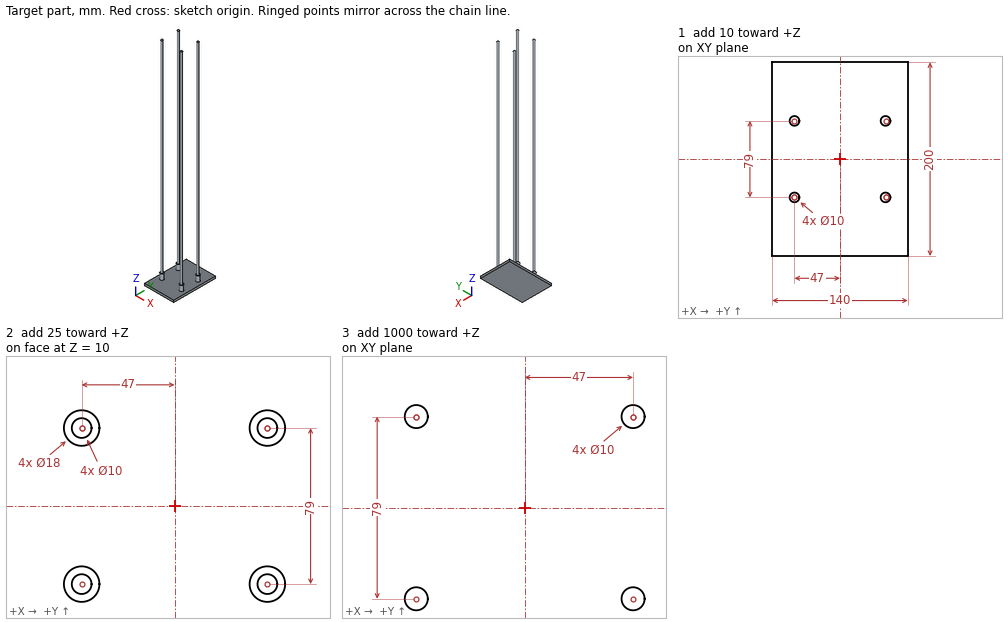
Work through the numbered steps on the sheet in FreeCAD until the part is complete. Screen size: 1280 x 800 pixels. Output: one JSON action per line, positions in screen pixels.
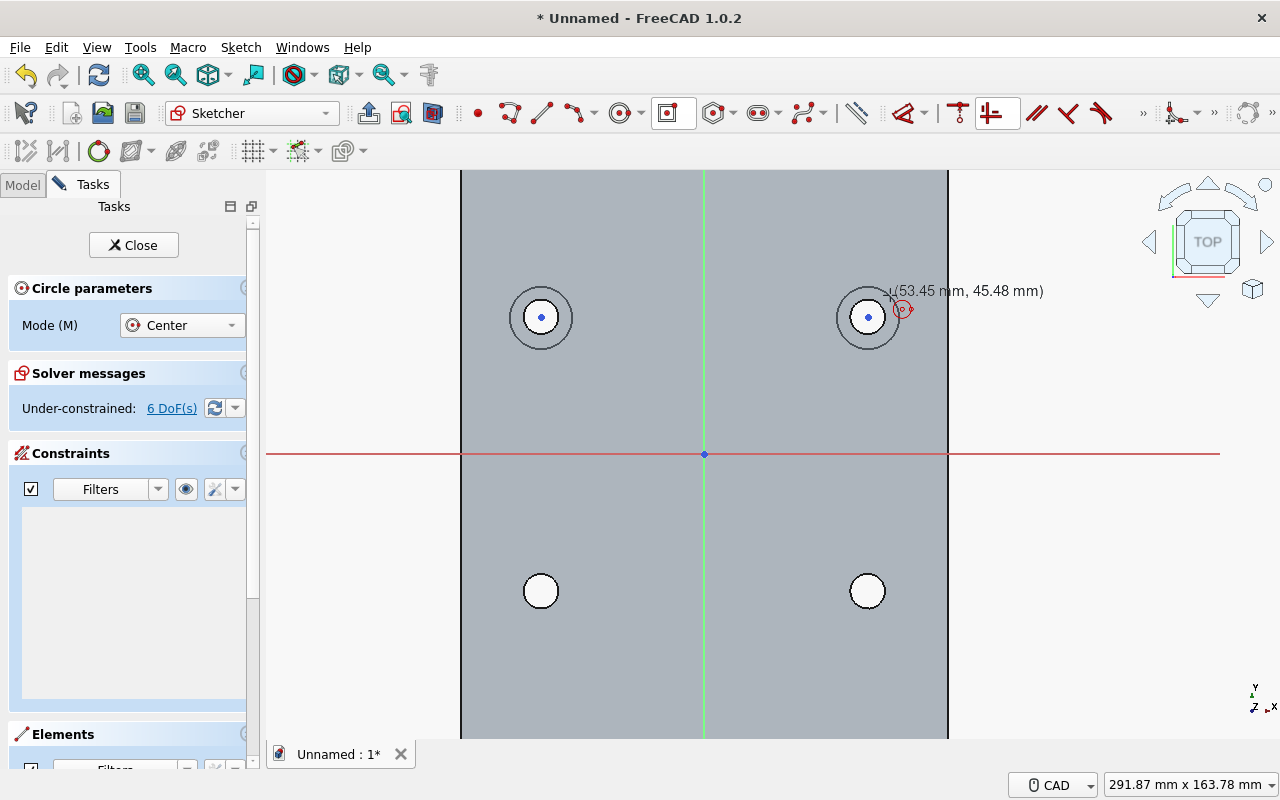
{"action": "left_click", "coordinate": [868, 591]}
{"action": "left_click", "coordinate": [890, 569]}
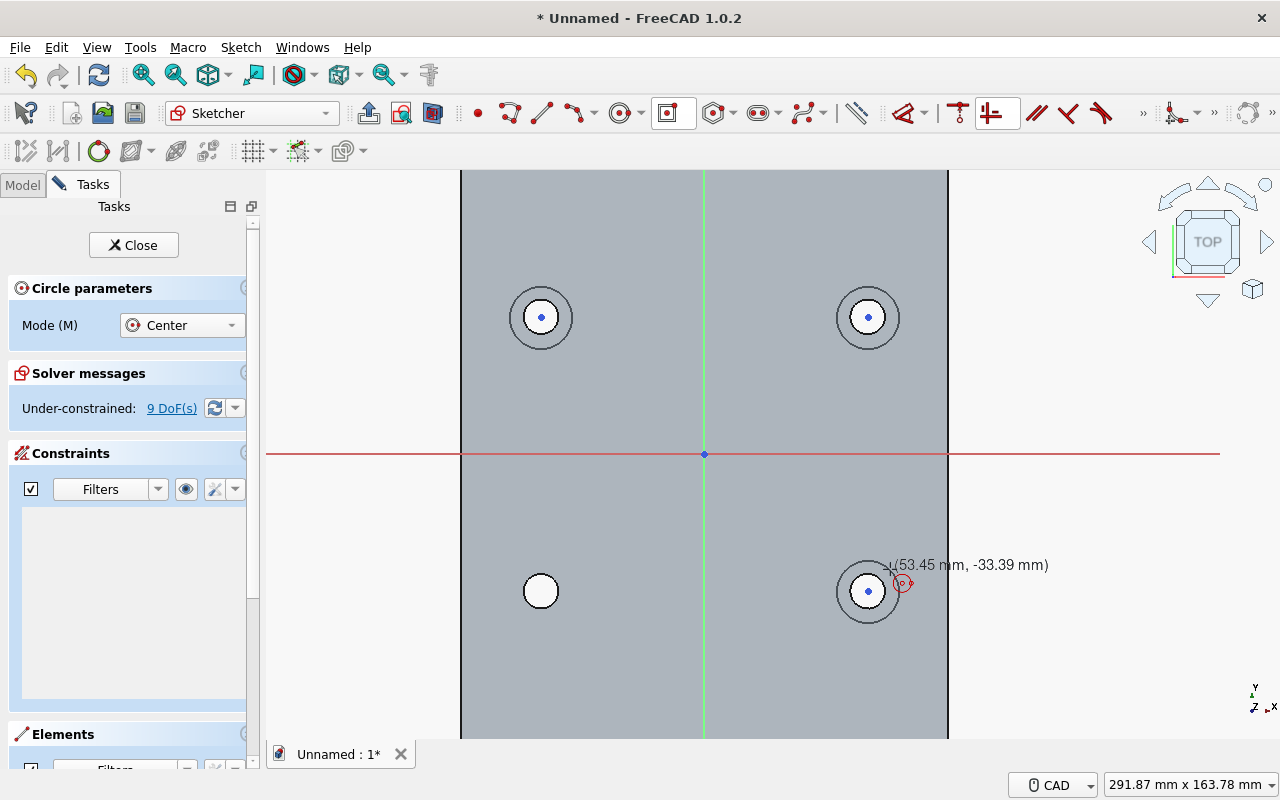
{"action": "left_click", "coordinate": [541, 591]}
{"action": "left_click", "coordinate": [563, 569]}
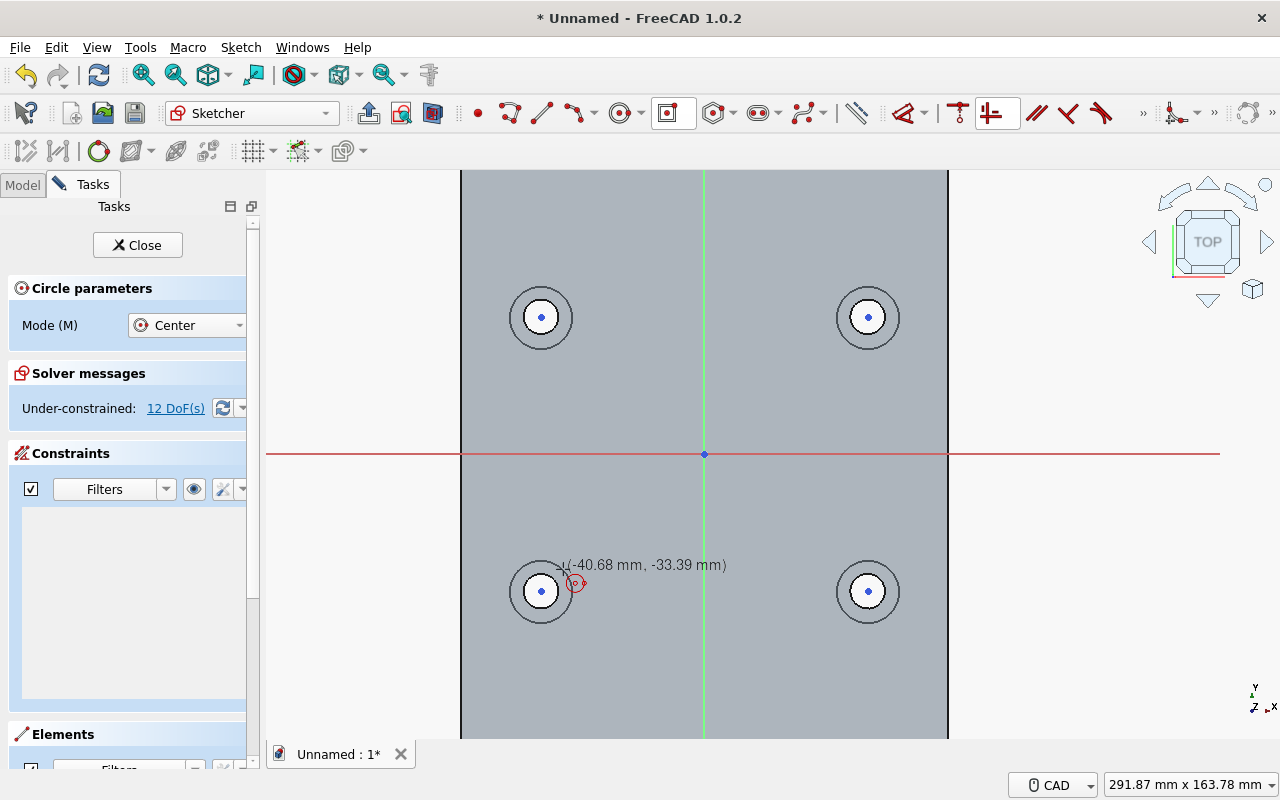
{"action": "scroll", "coordinate": [541, 317], "scroll_direction": "up", "scroll_amount": 2}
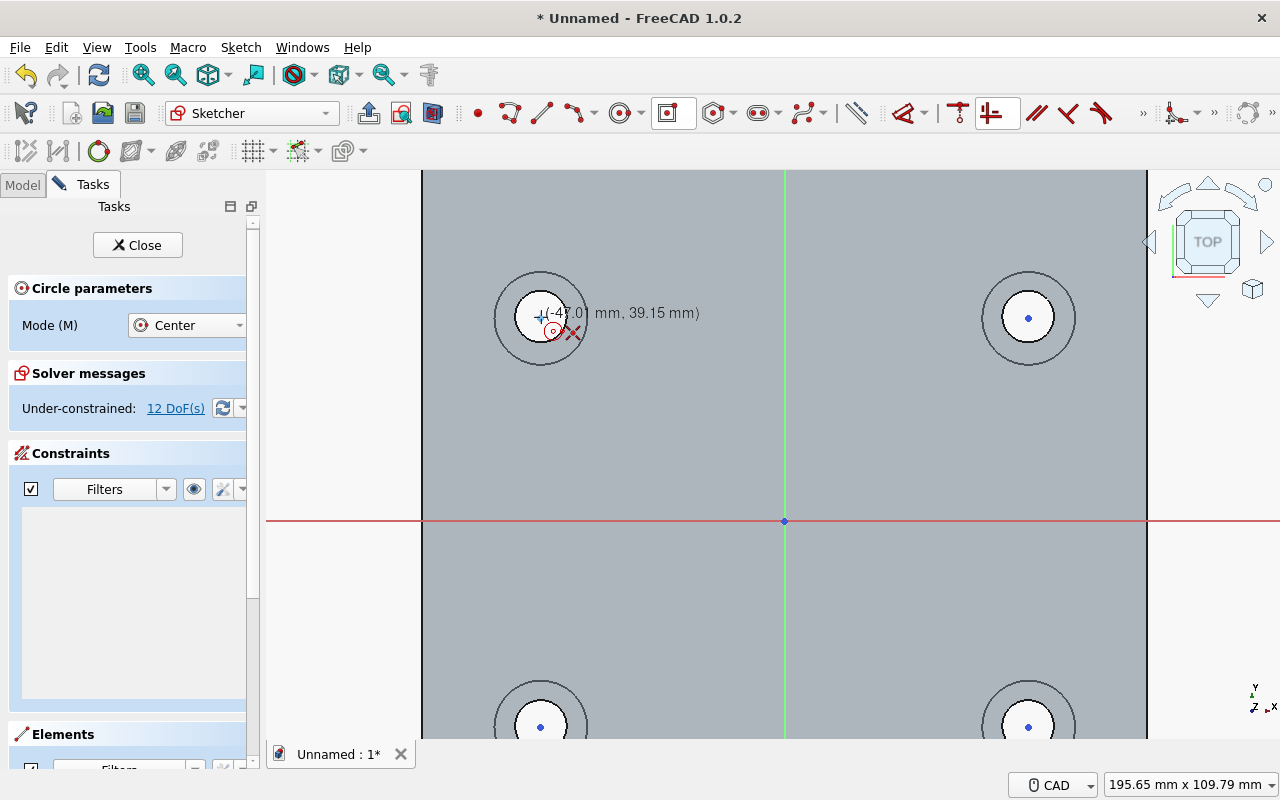
{"action": "left_click", "coordinate": [541, 318]}
{"action": "left_click", "coordinate": [559, 298]}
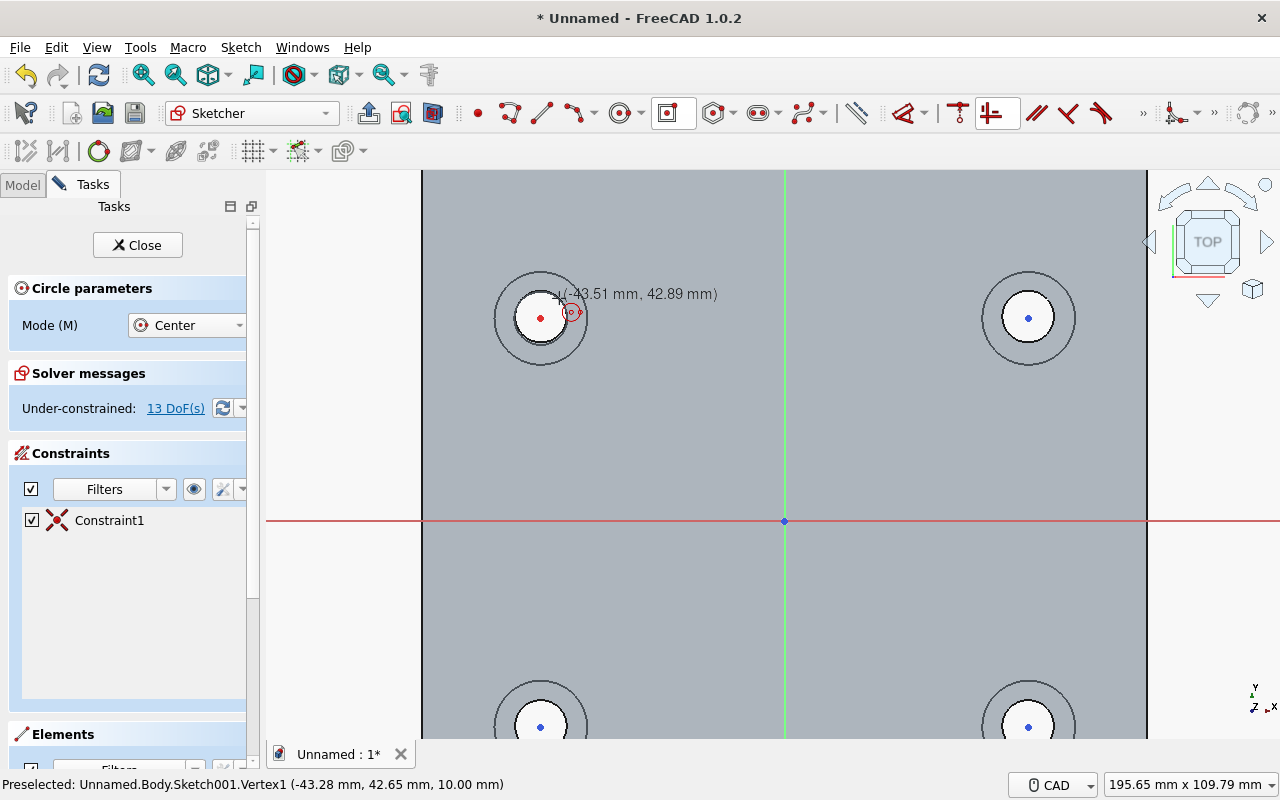
{"action": "left_click", "coordinate": [1029, 318]}
{"action": "left_click", "coordinate": [1046, 298]}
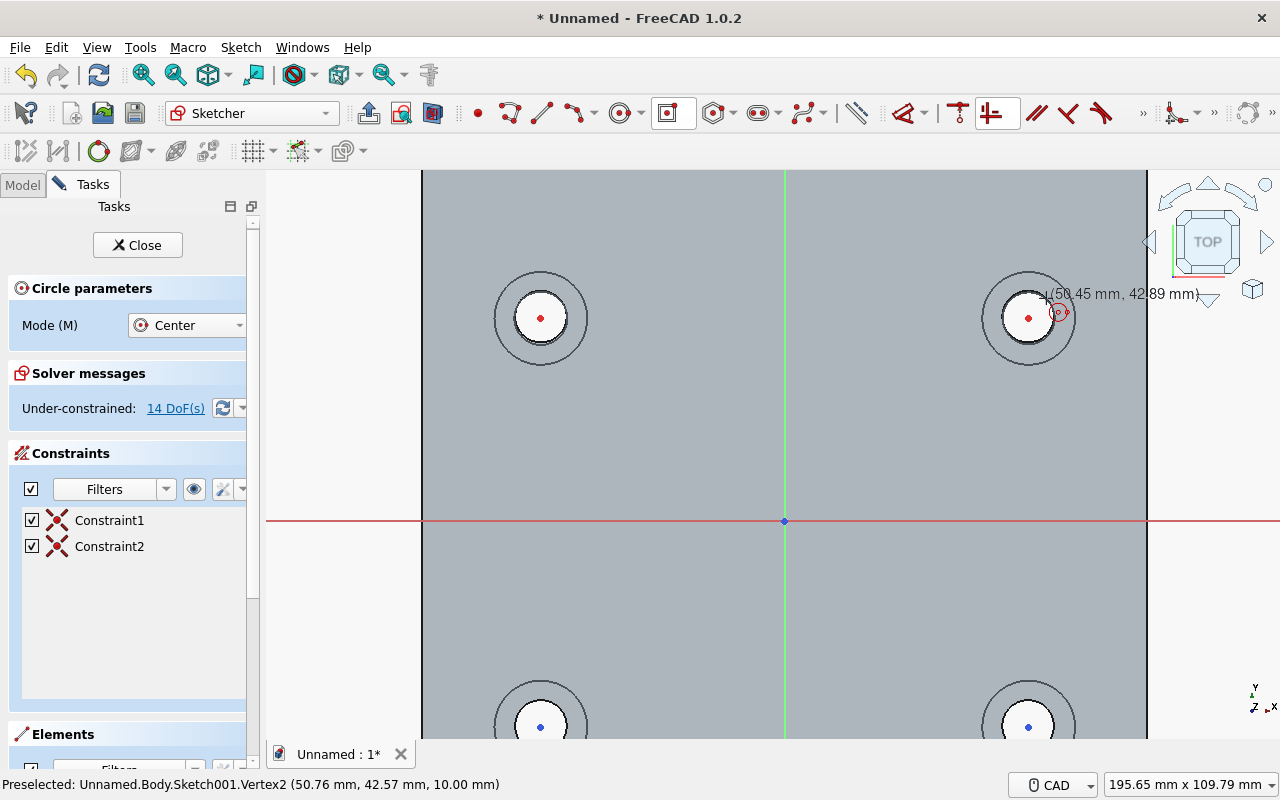
{"action": "scroll", "coordinate": [542, 319], "scroll_direction": "down", "scroll_amount": 2}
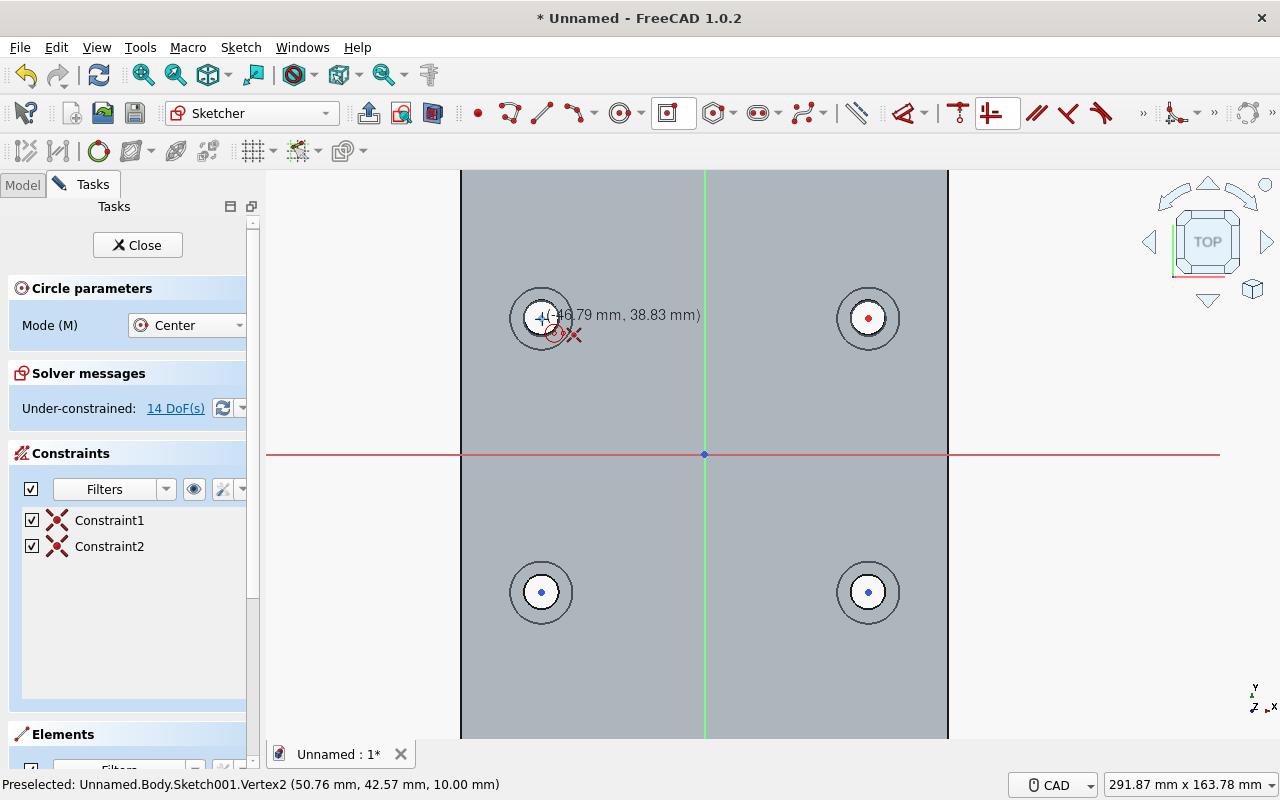
{"action": "scroll", "coordinate": [868, 592], "scroll_direction": "up", "scroll_amount": 2}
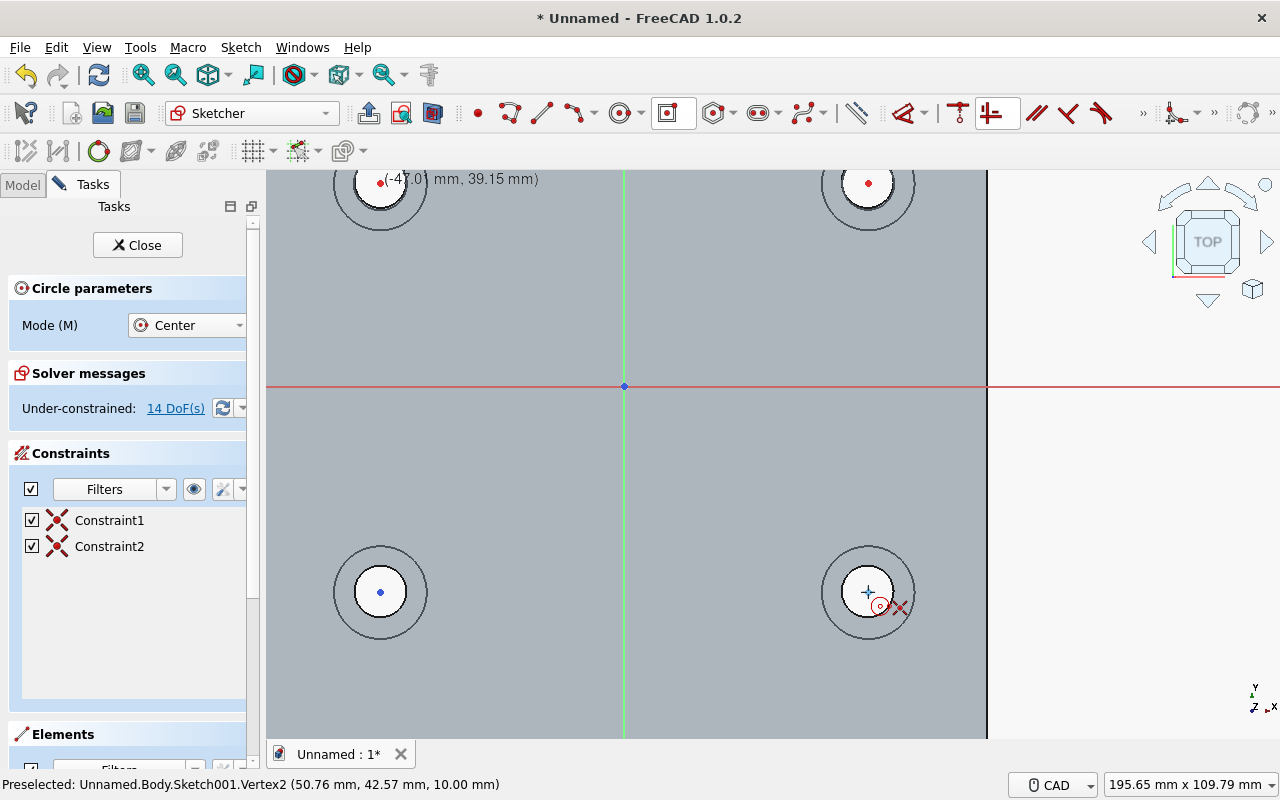
{"action": "left_click", "coordinate": [868, 593]}
{"action": "left_click", "coordinate": [886, 573]}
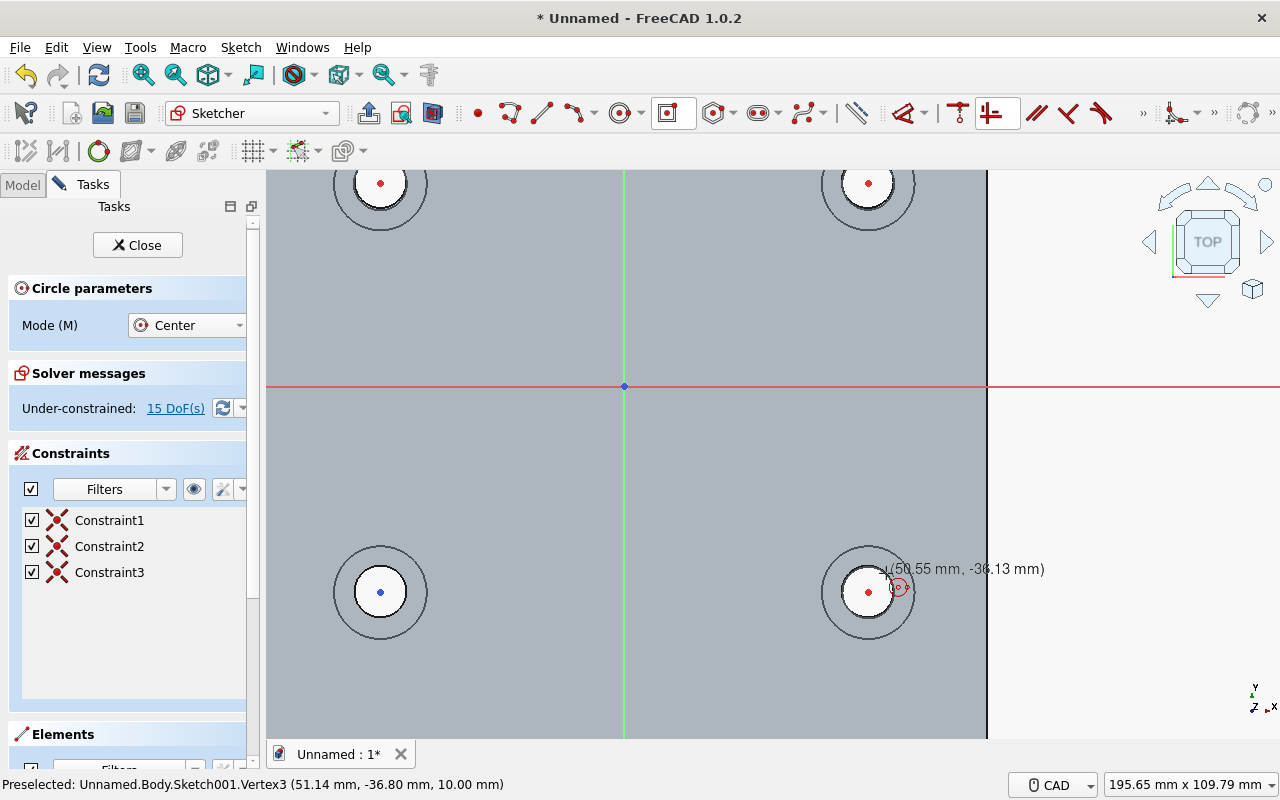
{"action": "left_click", "coordinate": [380, 593]}
{"action": "left_click", "coordinate": [399, 573]}
{"action": "key", "text": "Escape"}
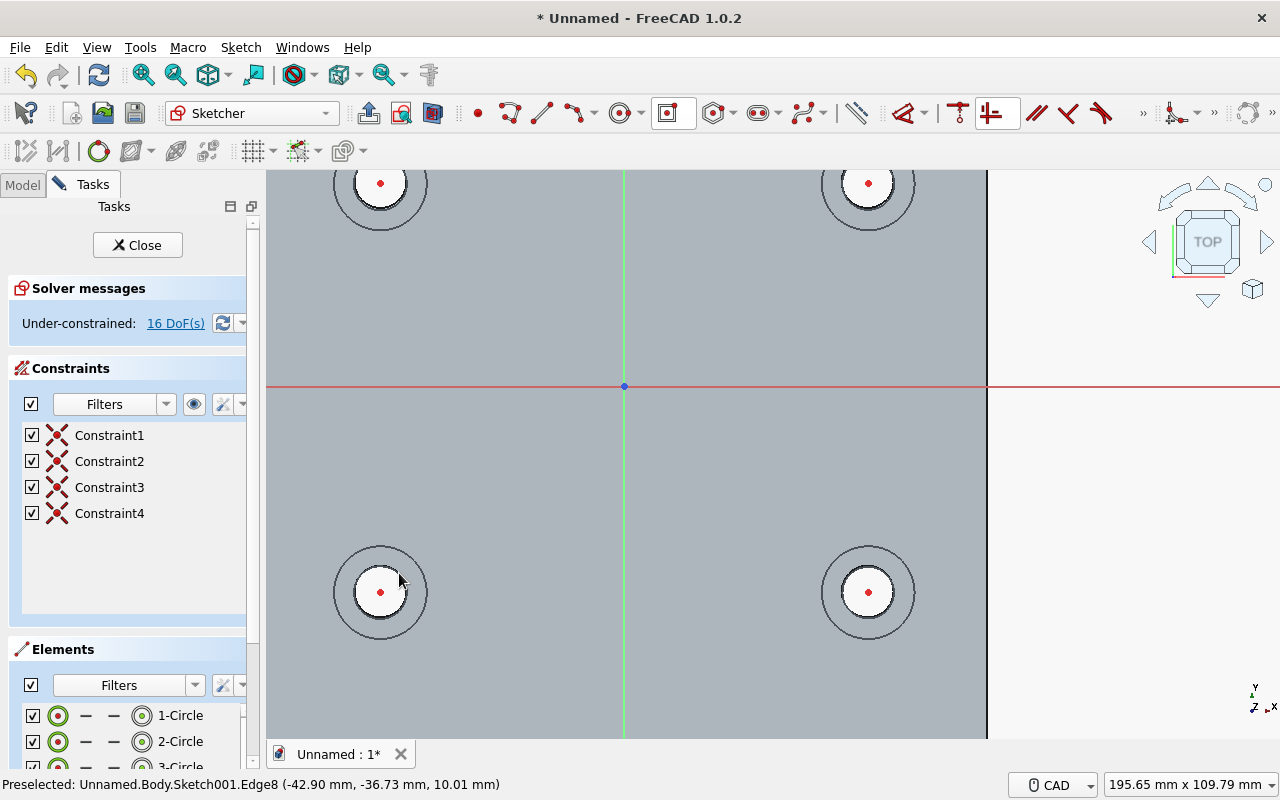
{"action": "left_click", "coordinate": [348, 217]}